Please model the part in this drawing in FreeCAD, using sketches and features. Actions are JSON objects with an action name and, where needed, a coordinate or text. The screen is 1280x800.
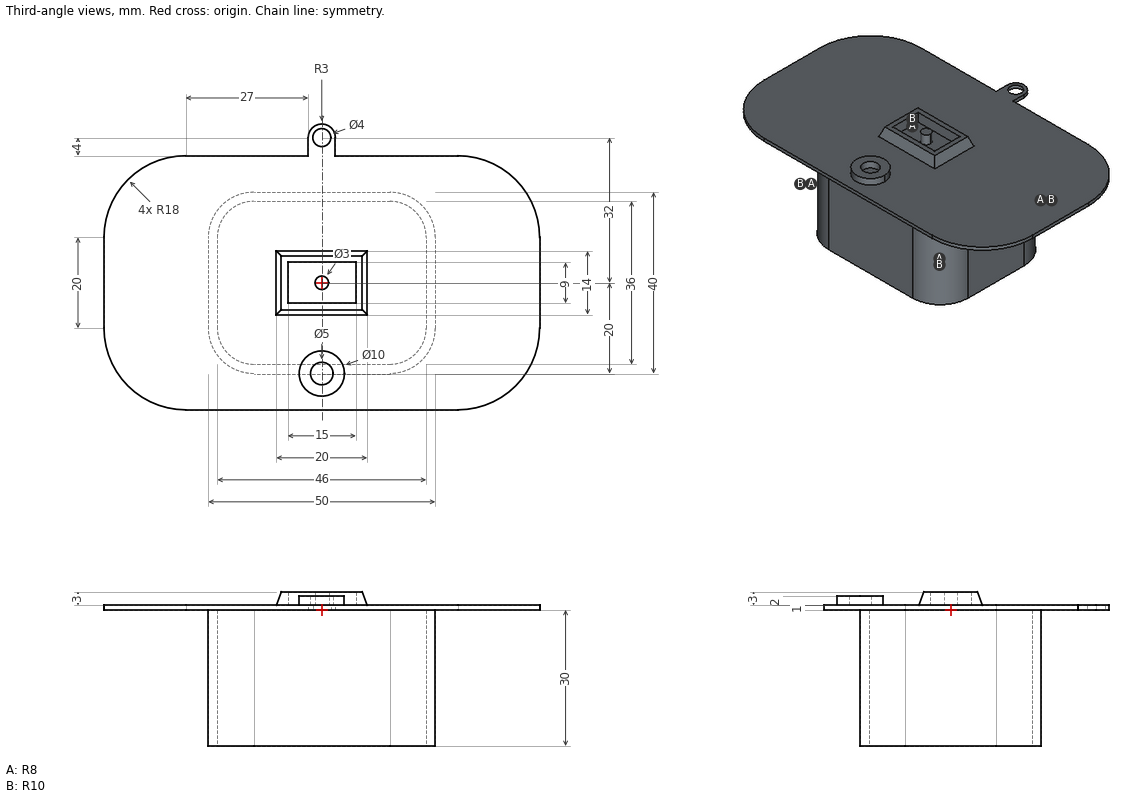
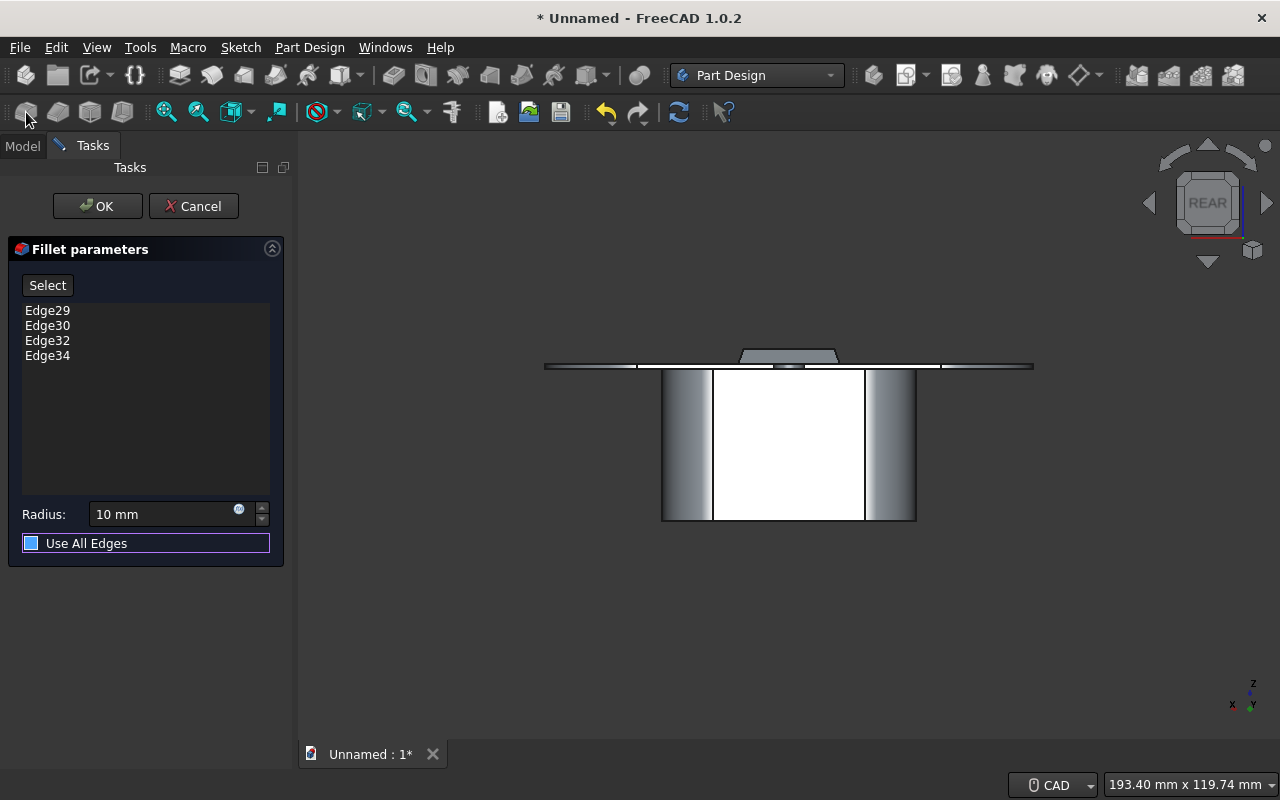
{"action": "left_click", "coordinate": [98, 206]}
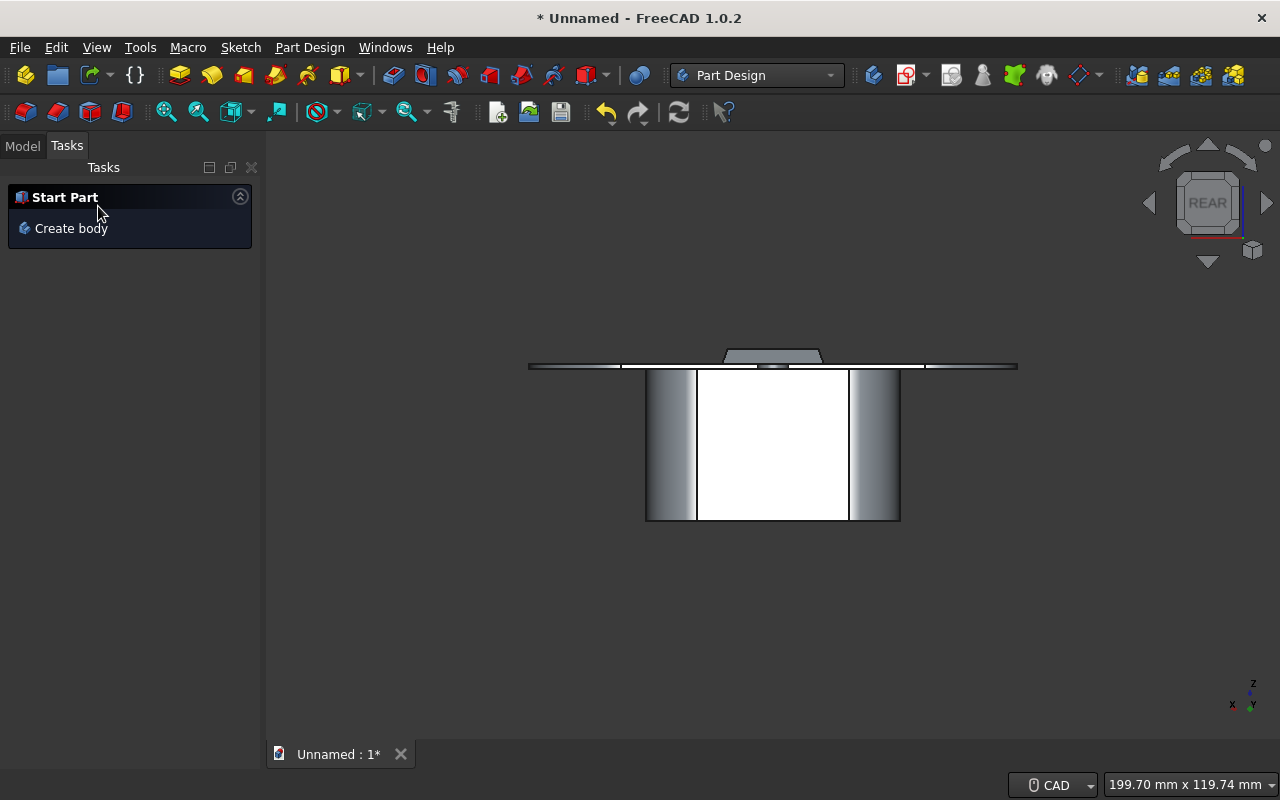
{"action": "key", "text": "0"}